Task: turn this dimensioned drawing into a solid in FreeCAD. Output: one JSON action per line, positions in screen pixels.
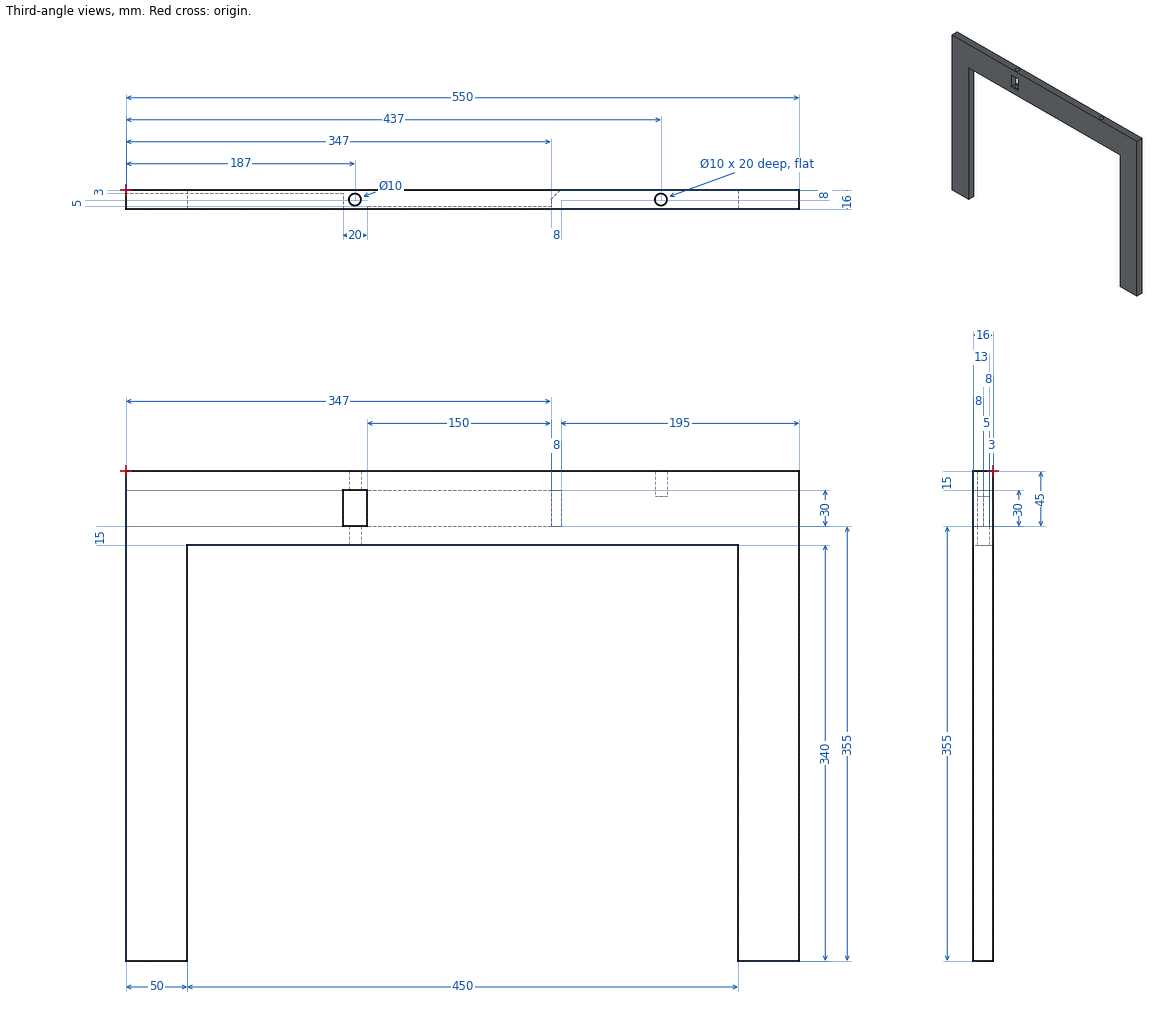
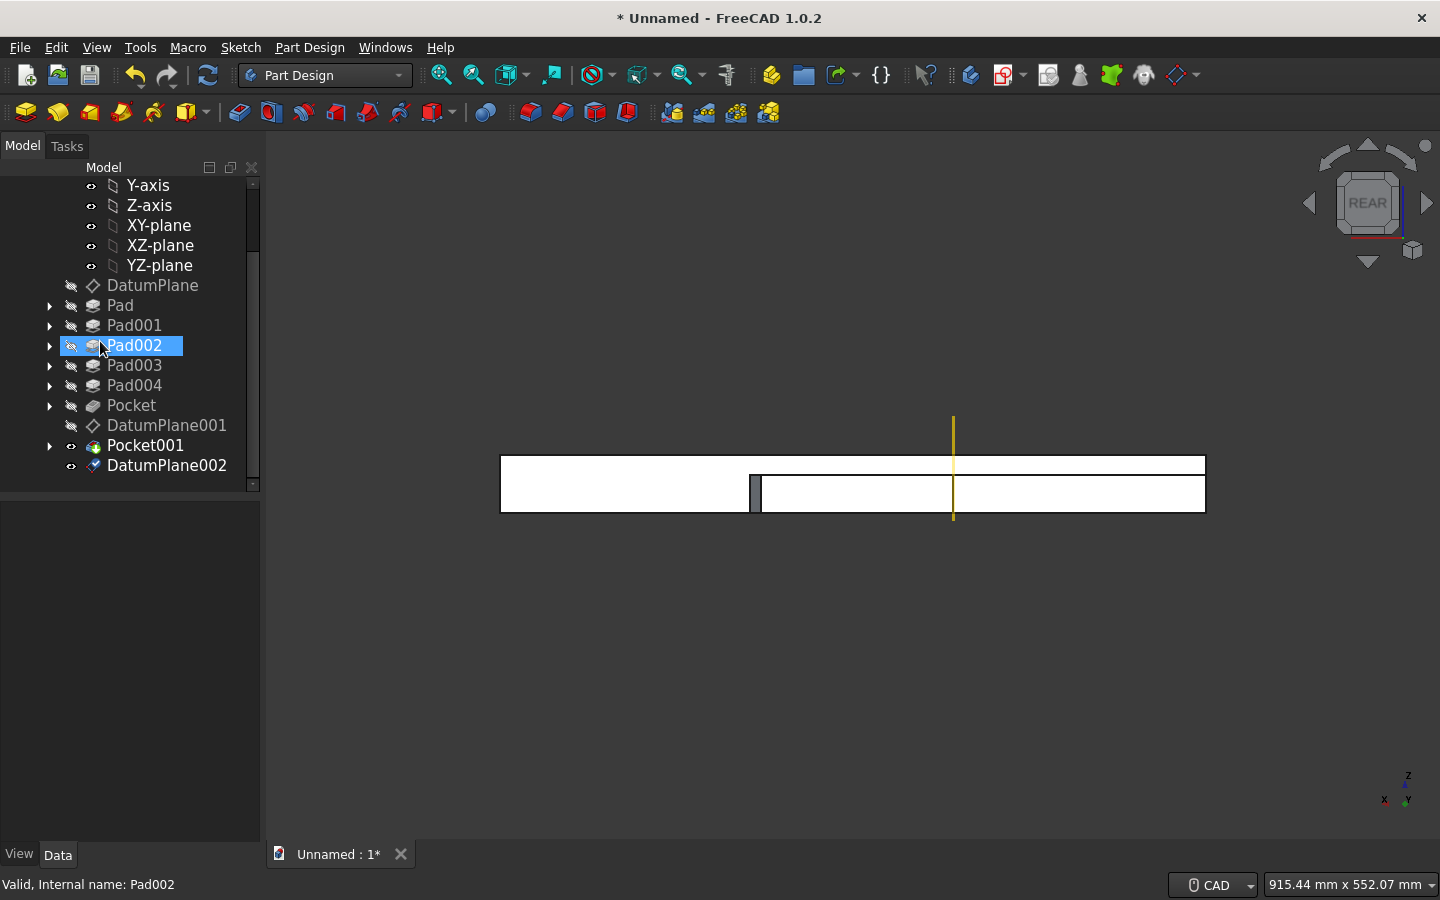
{"action": "left_click", "coordinate": [116, 466]}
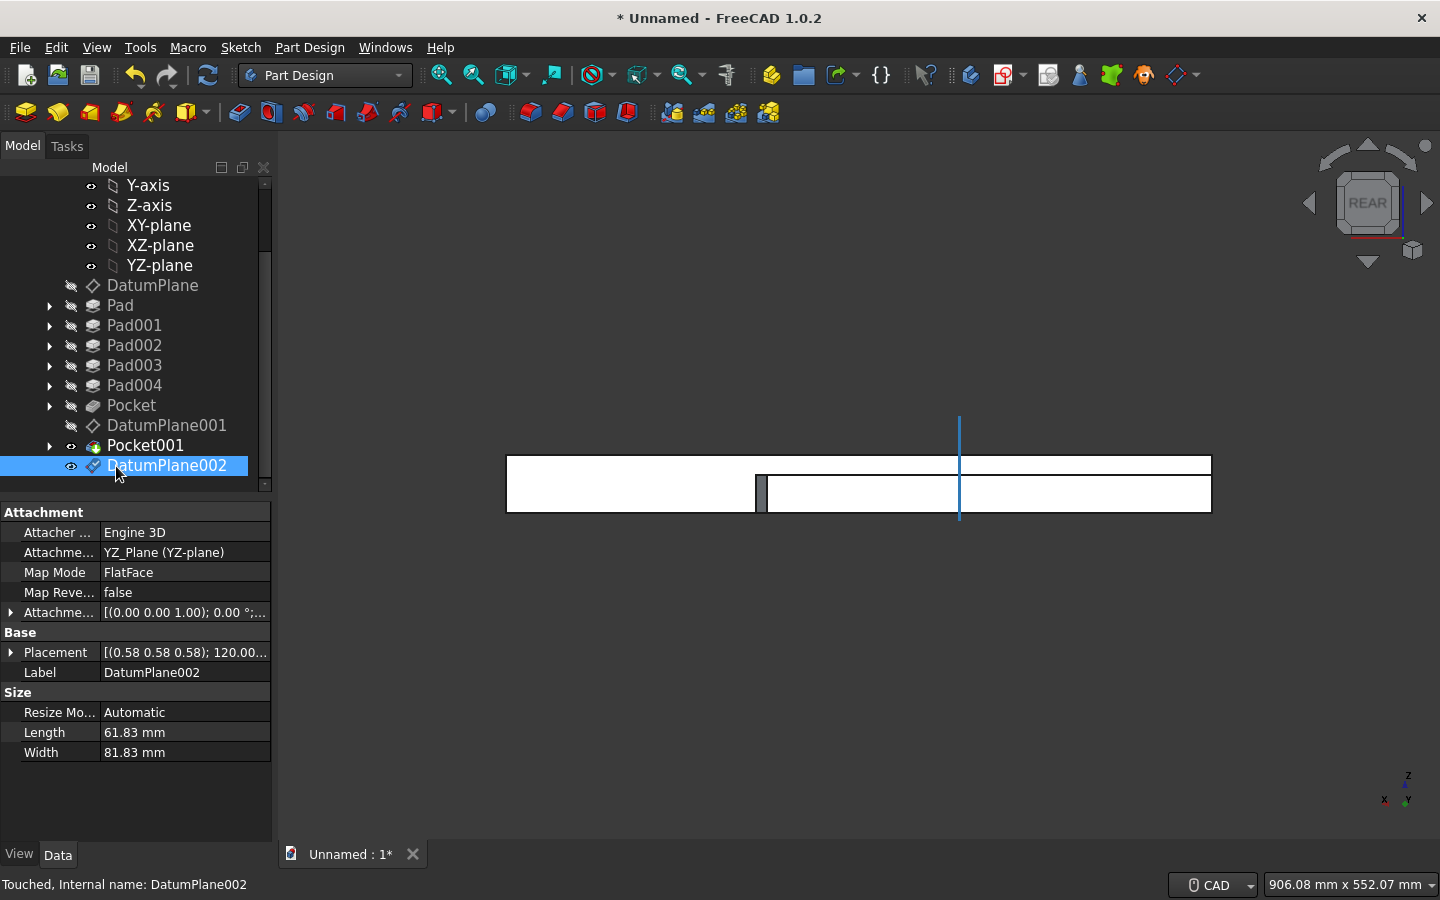
{"action": "left_click", "coordinate": [1004, 76]}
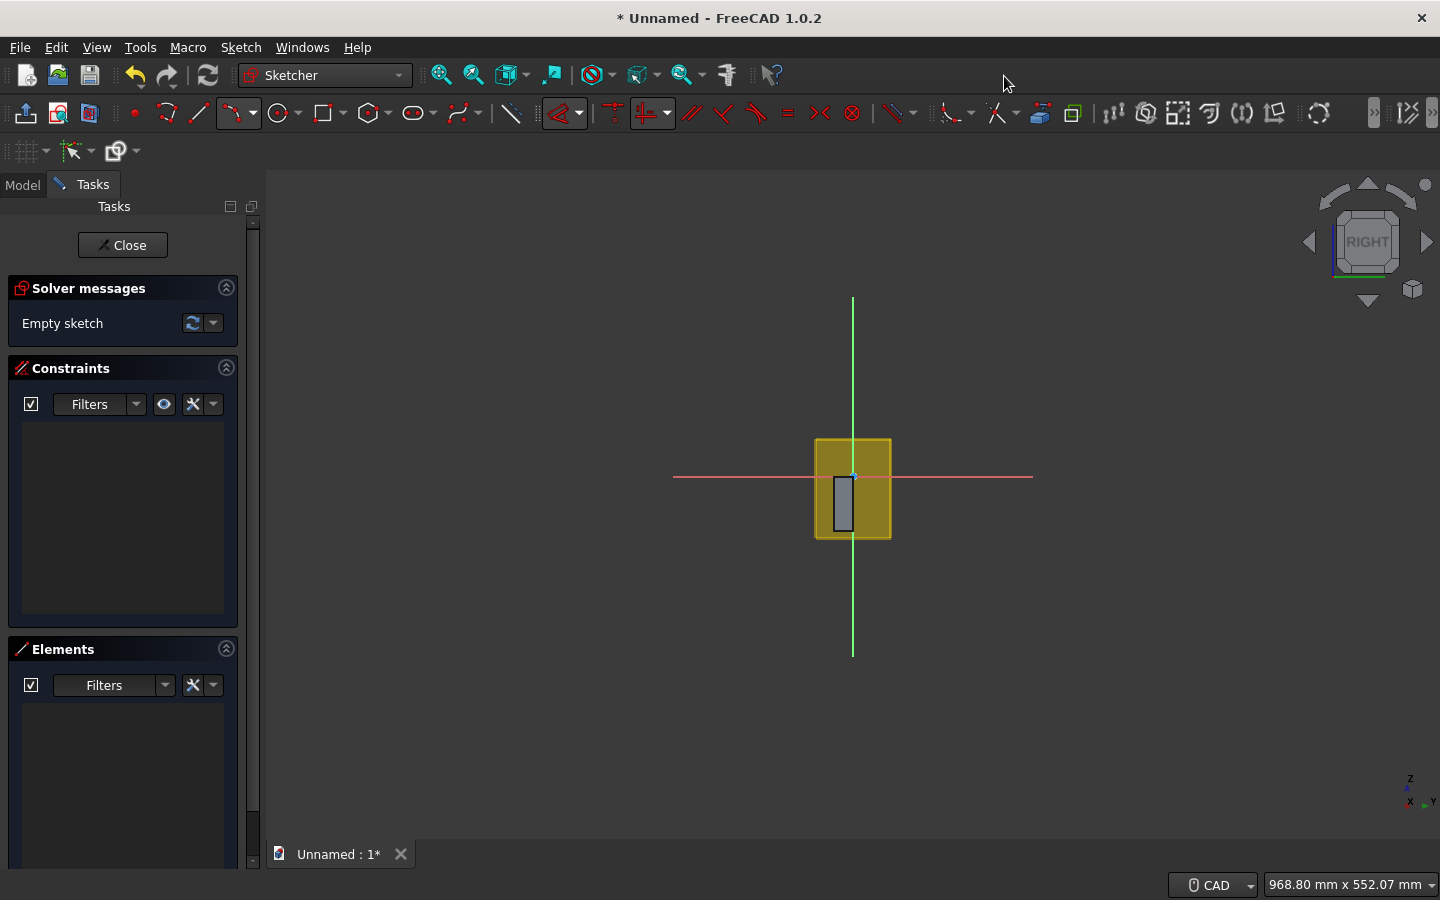
{"action": "left_click", "coordinate": [90, 114]}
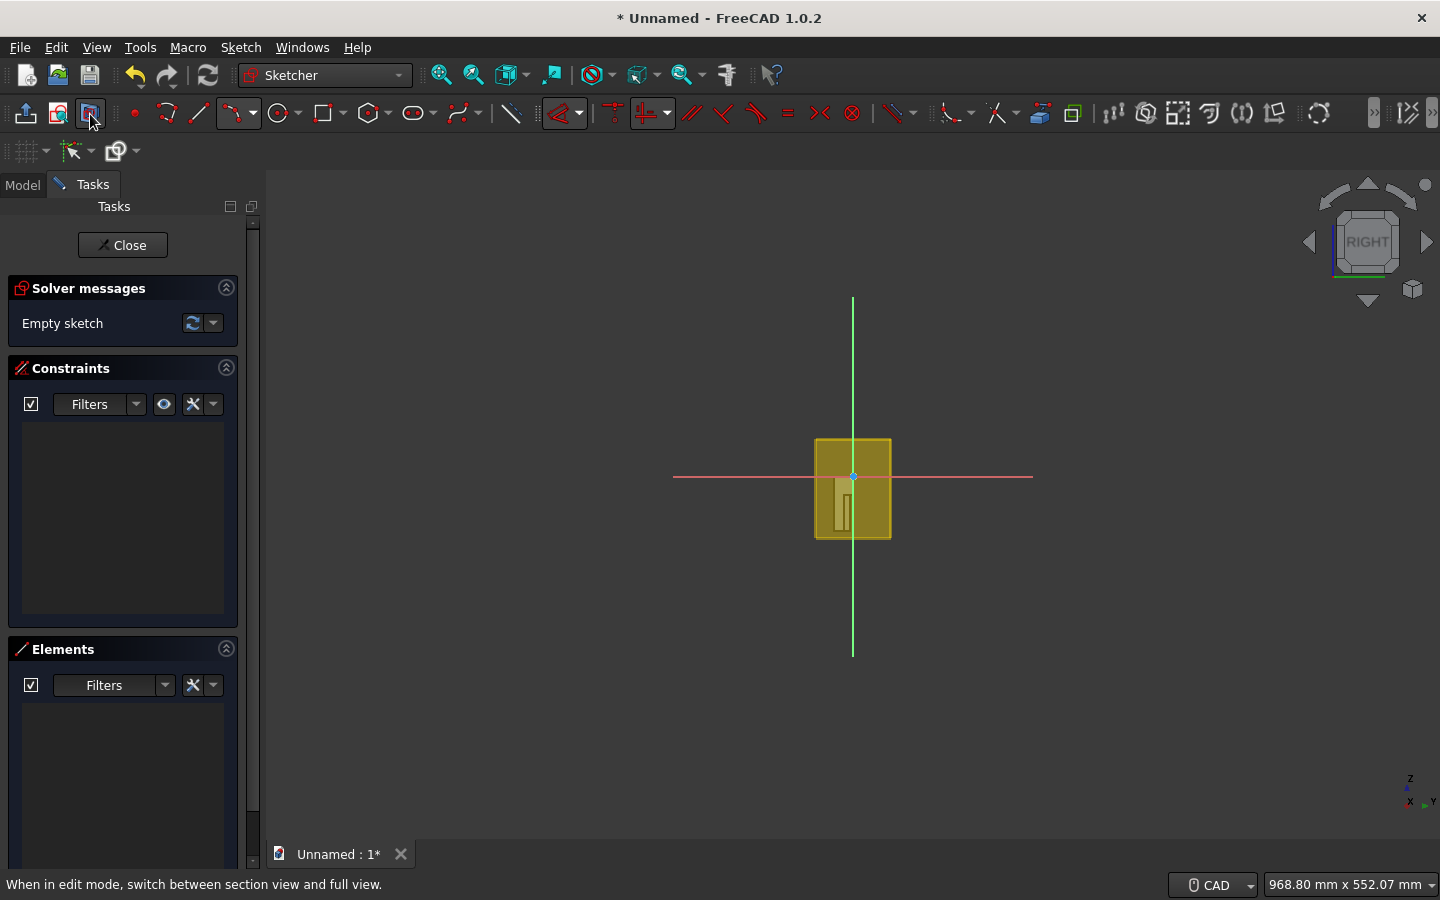
{"action": "scroll", "coordinate": [853, 504], "scroll_direction": "up", "scroll_amount": 10}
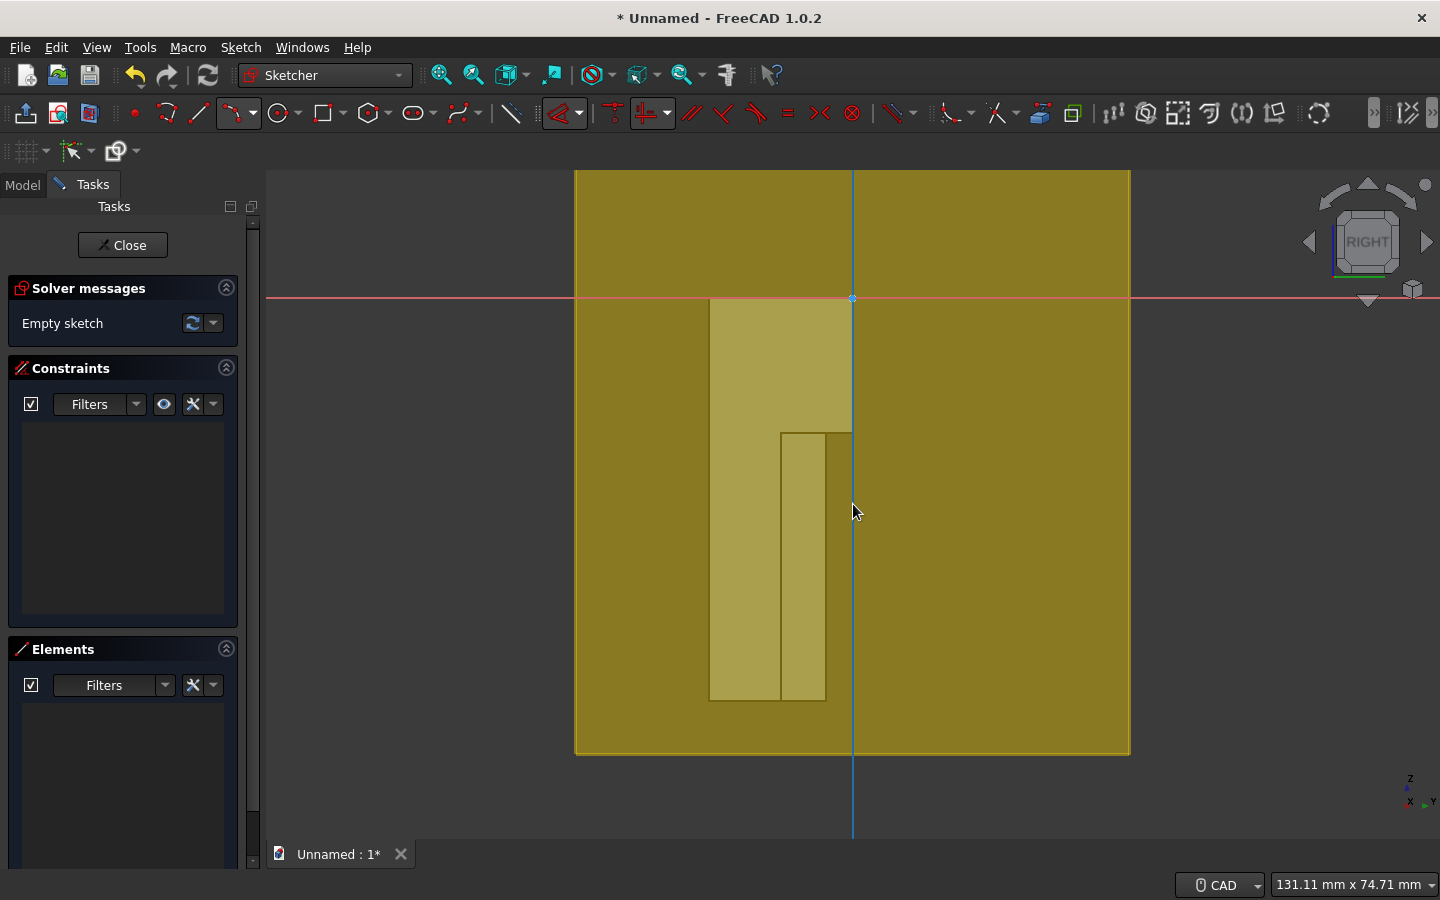
{"action": "left_click", "coordinate": [324, 114]}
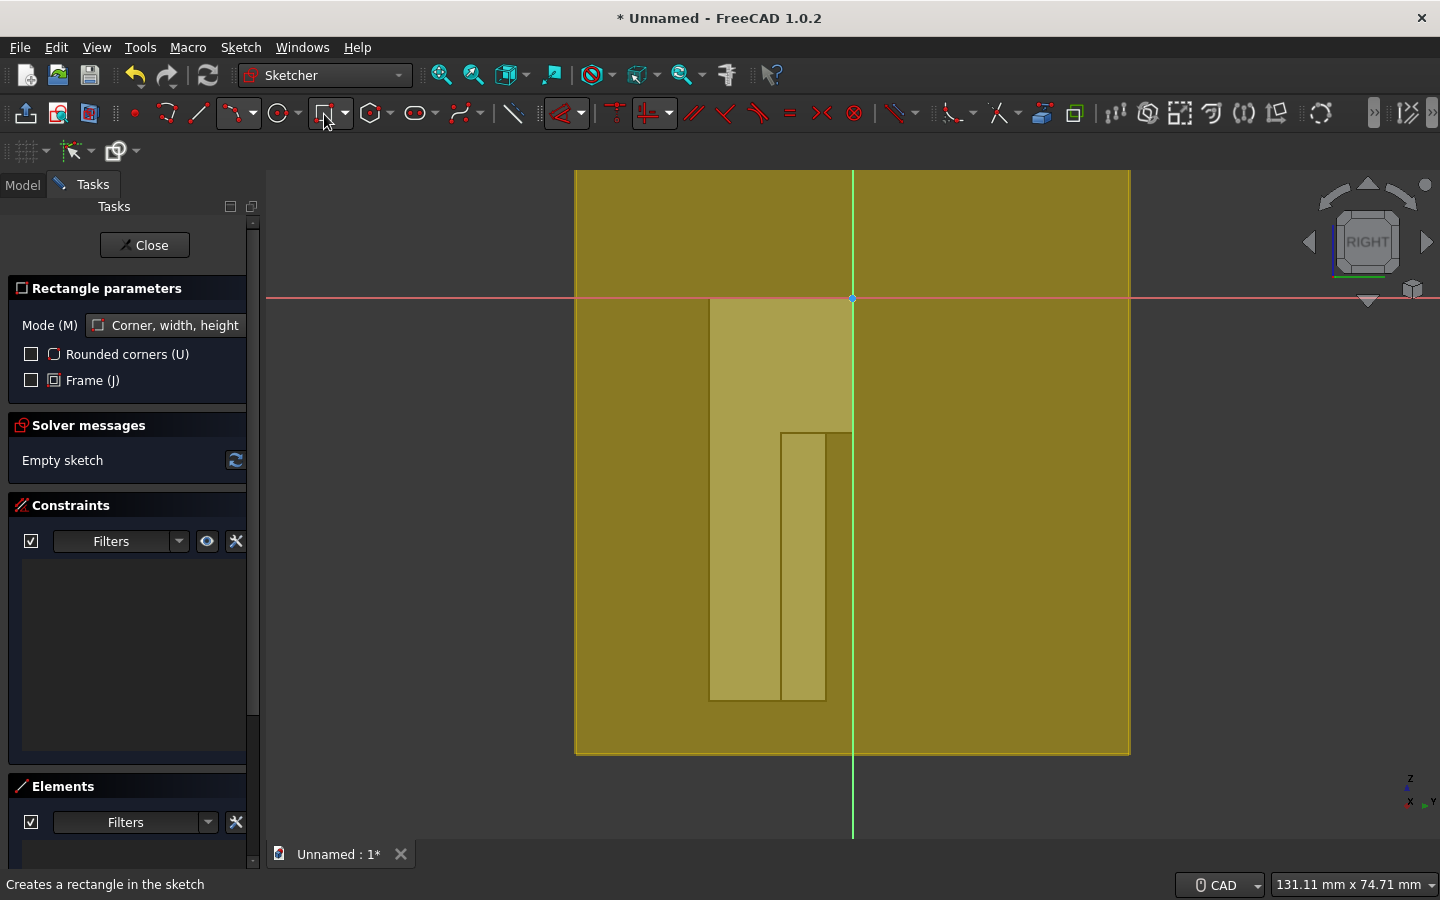
{"action": "left_click", "coordinate": [709, 433]}
{"action": "left_click", "coordinate": [826, 701]}
{"action": "key", "text": "Escape"}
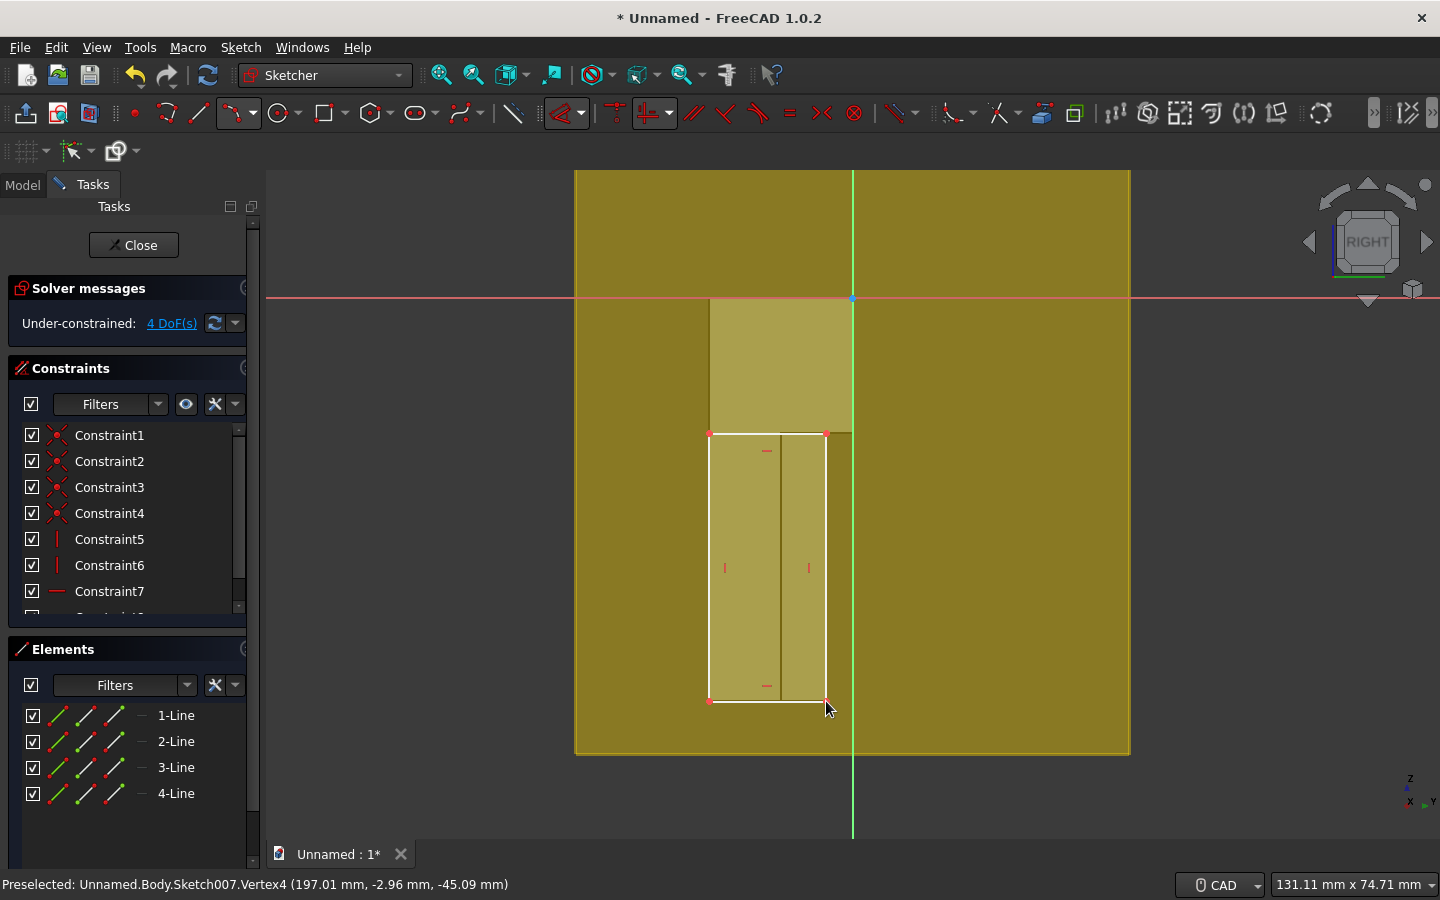
{"action": "left_click", "coordinate": [709, 514]}